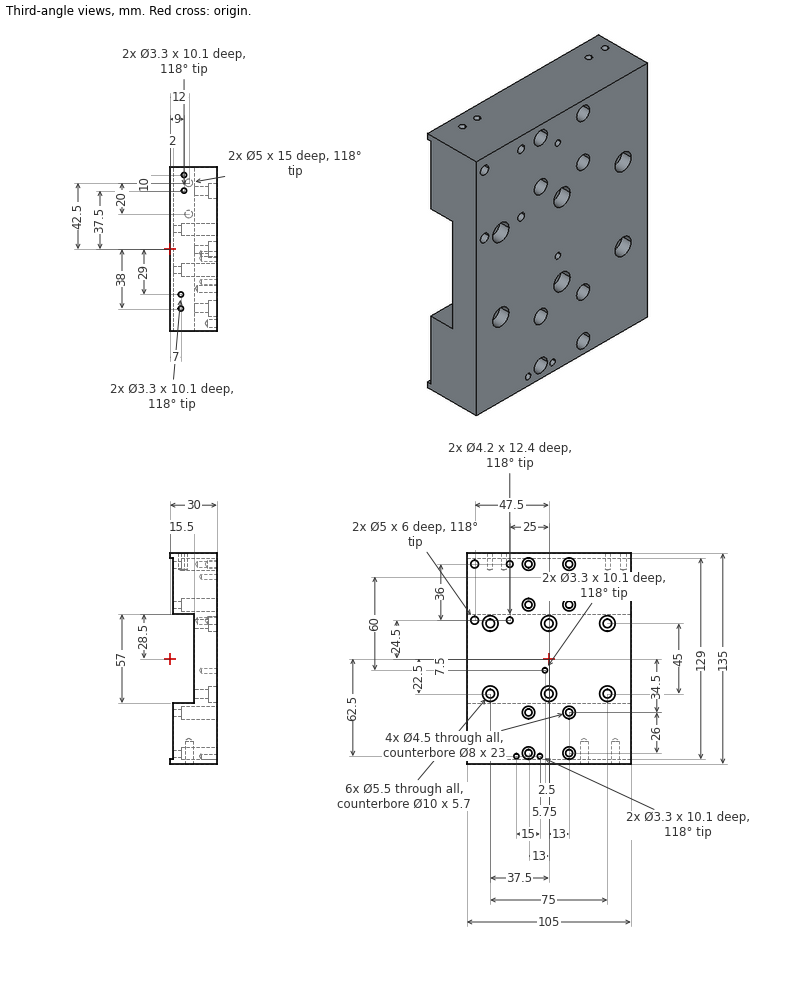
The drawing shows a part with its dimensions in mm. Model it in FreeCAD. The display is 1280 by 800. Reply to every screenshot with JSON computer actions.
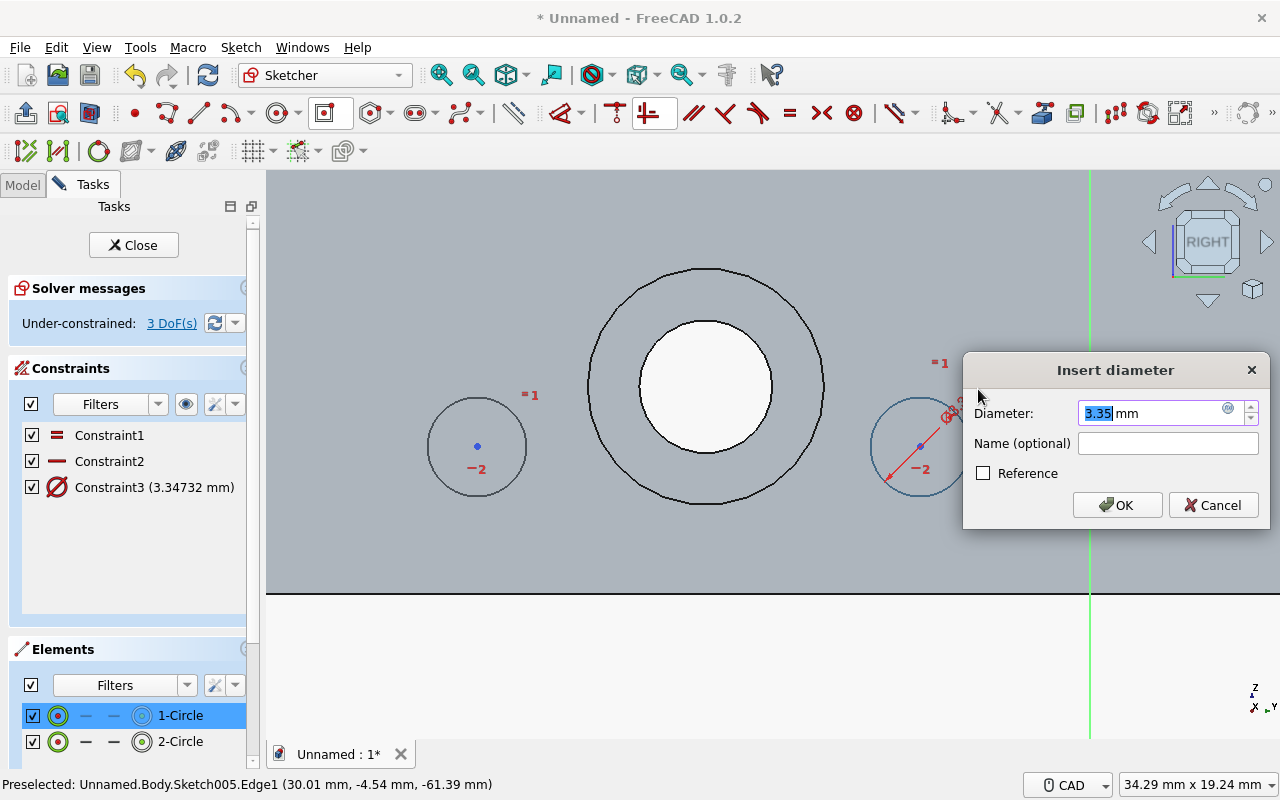
{"action": "type", "text": "3.3"}
{"action": "key", "text": "Return"}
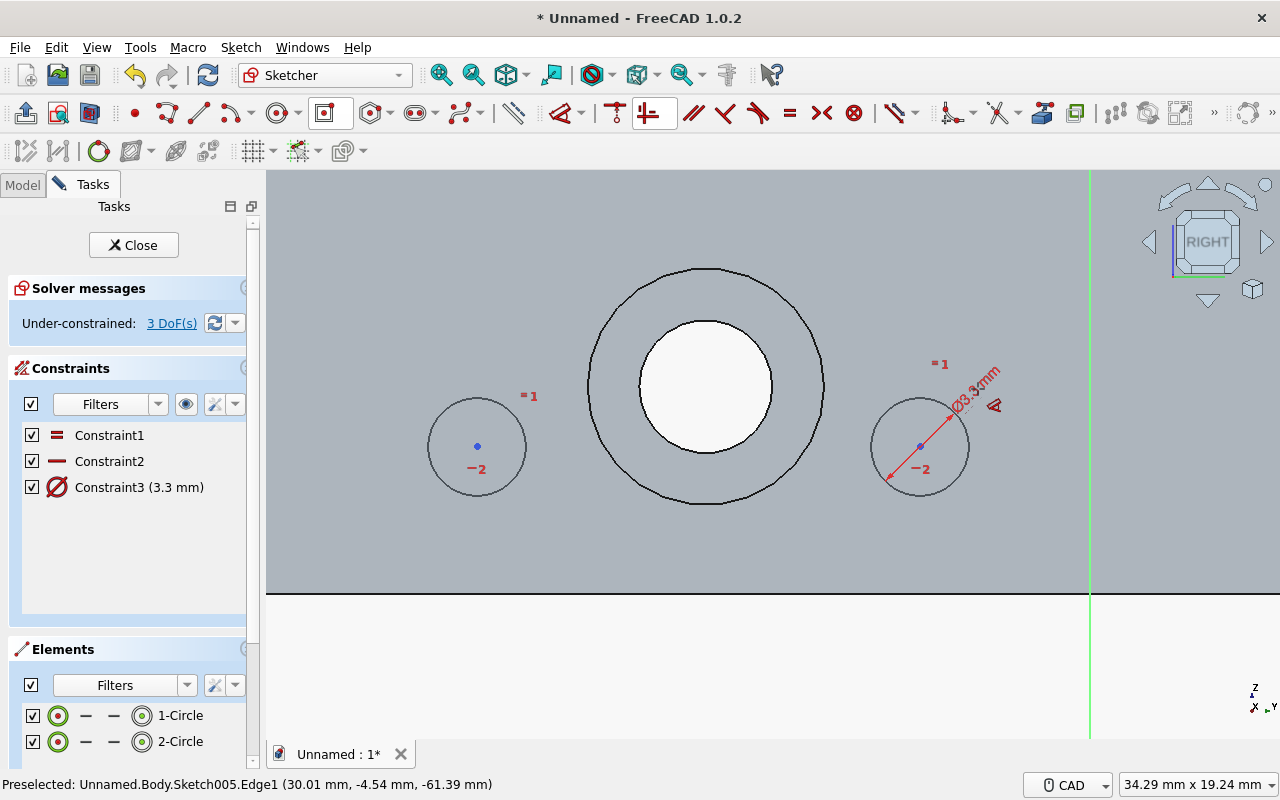
{"action": "left_click", "coordinate": [920, 447]}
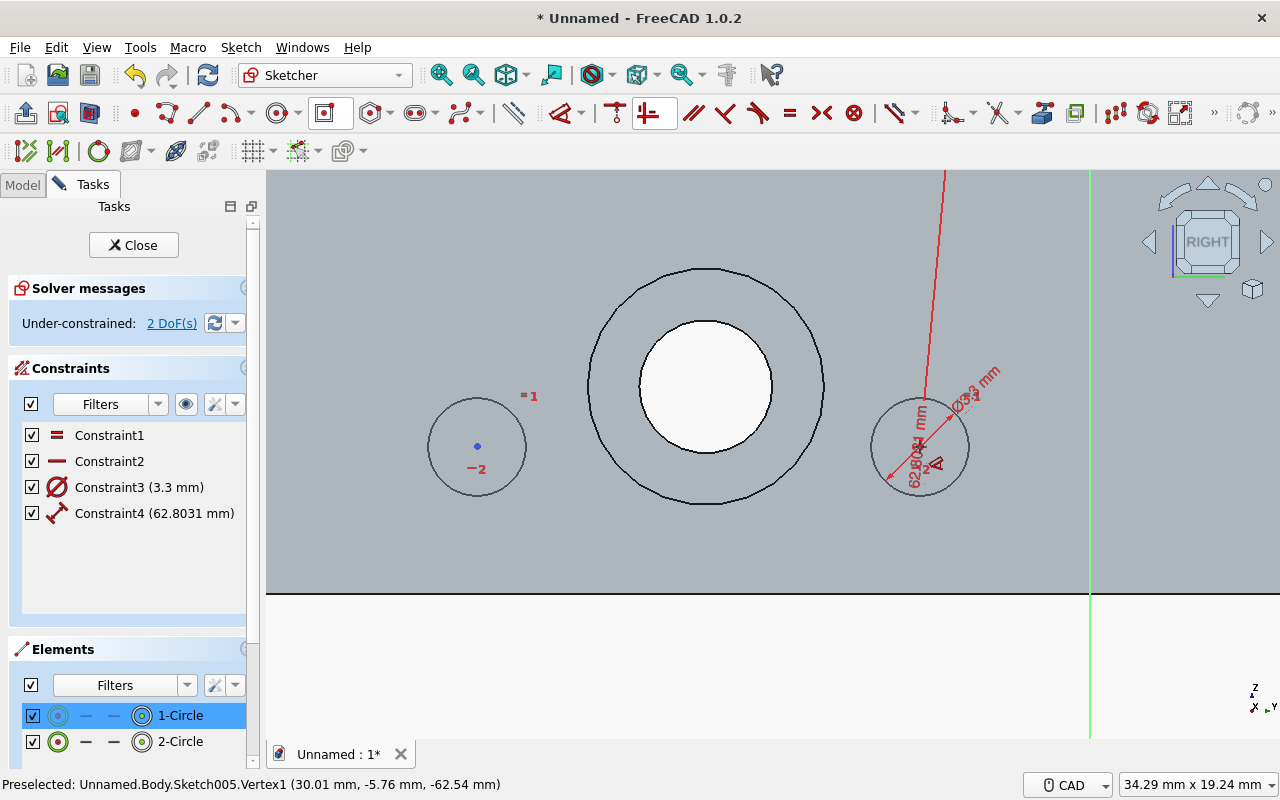
{"action": "left_click", "coordinate": [477, 447]}
{"action": "left_click", "coordinate": [699, 481]}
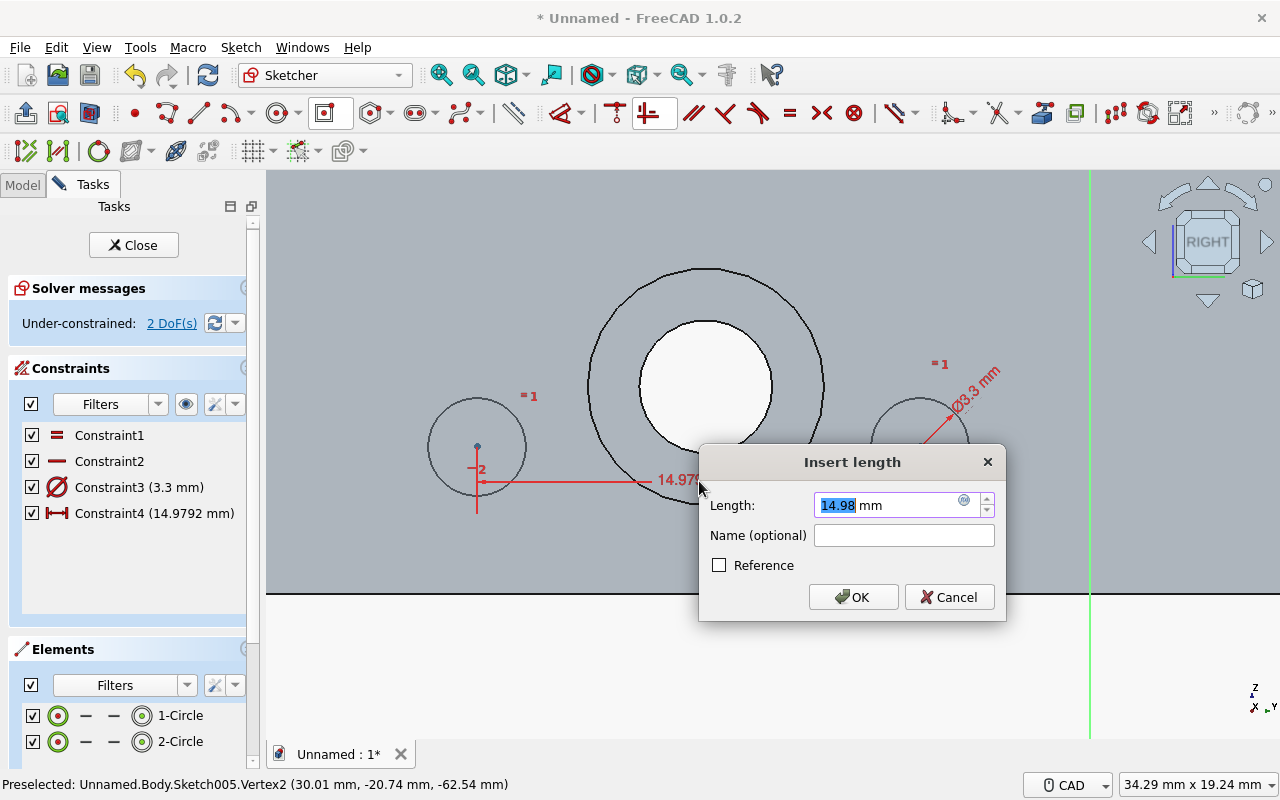
{"action": "type", "text": "15"}
{"action": "key", "text": "Return"}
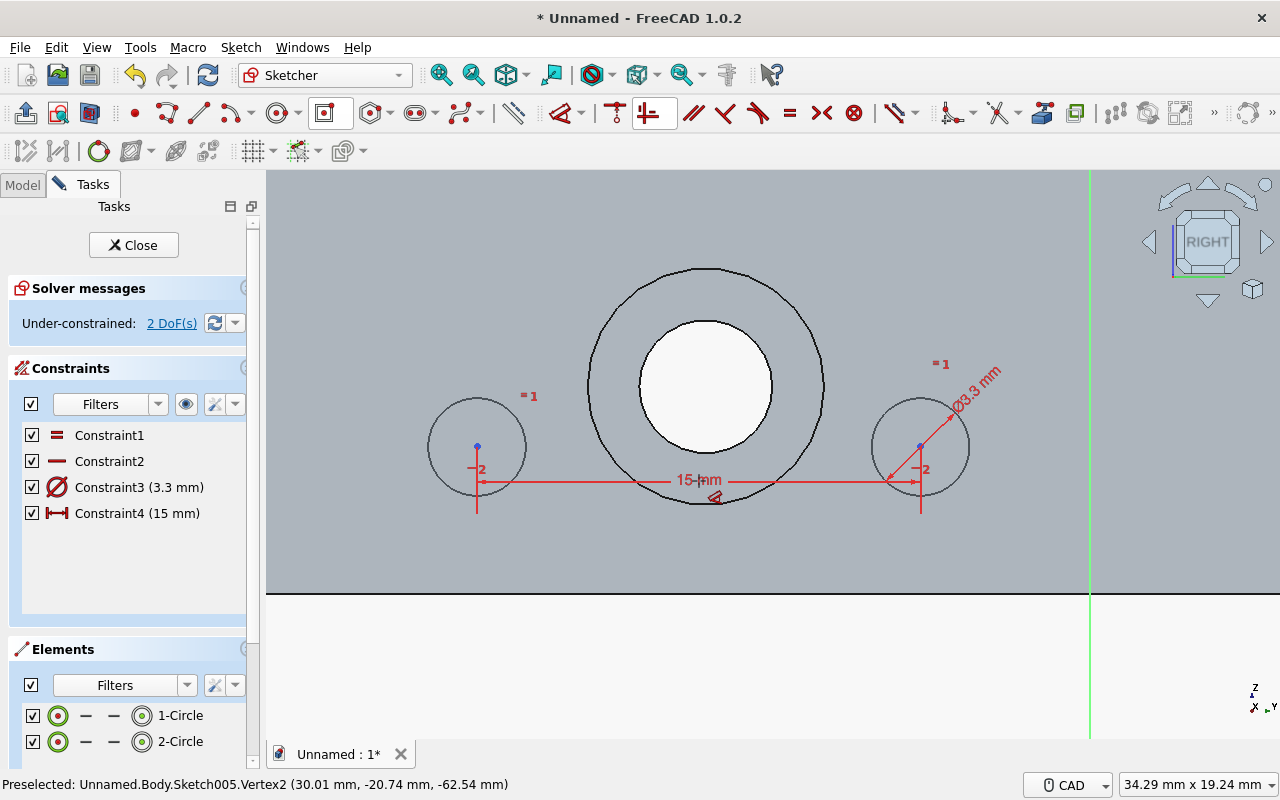
{"action": "left_click", "coordinate": [921, 447]}
{"action": "left_click", "coordinate": [1005, 481]}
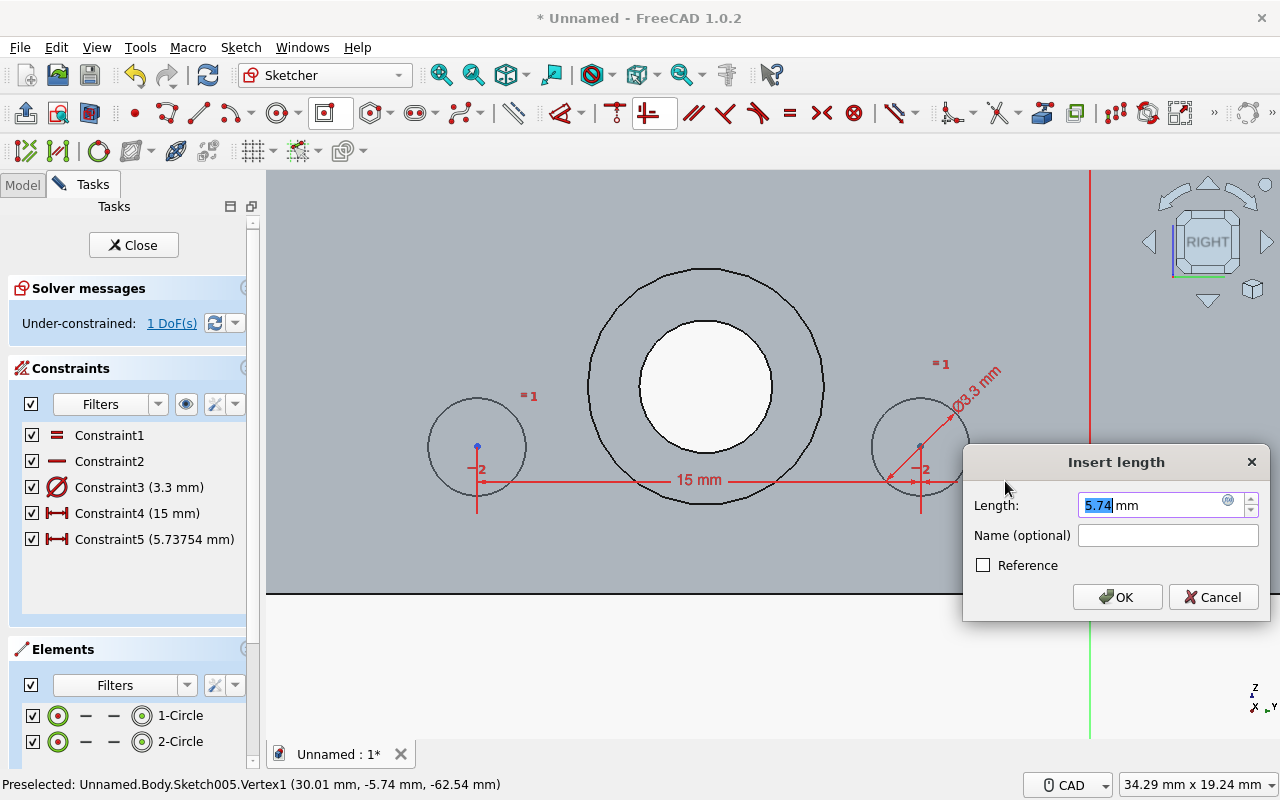
{"action": "type", "text": "5.75"}
{"action": "key", "text": "Return"}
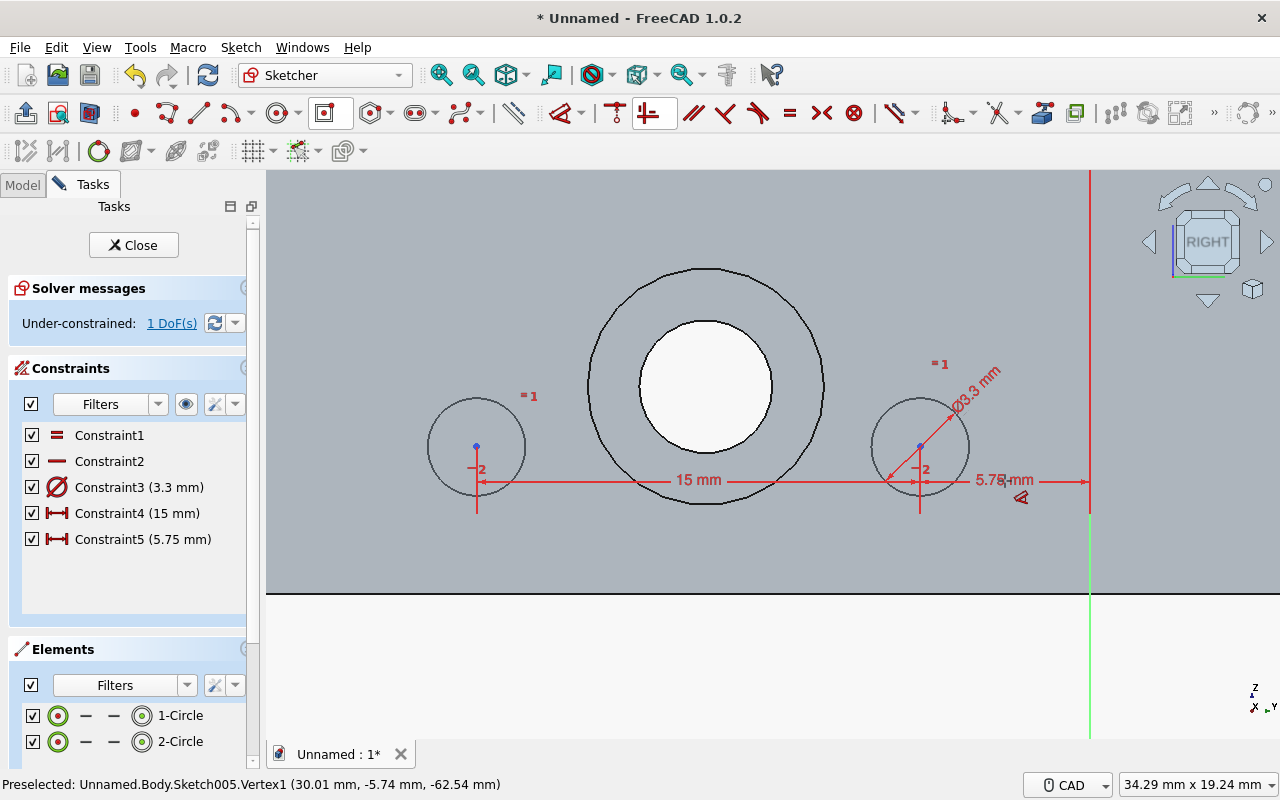
{"action": "left_click", "coordinate": [920, 447]}
{"action": "left_click", "coordinate": [886, 322]}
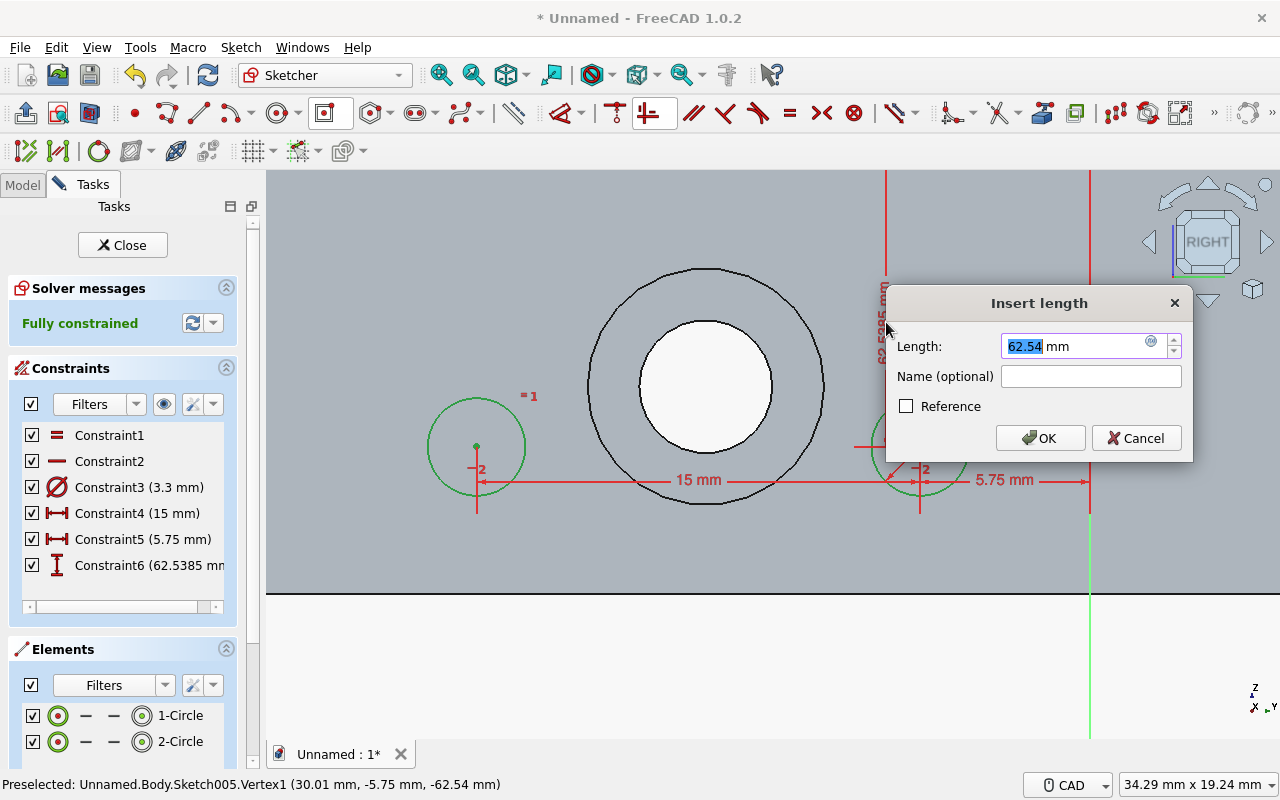
{"action": "type", "text": "62.5"}
{"action": "key", "text": "Return"}
{"action": "key", "text": "Escape"}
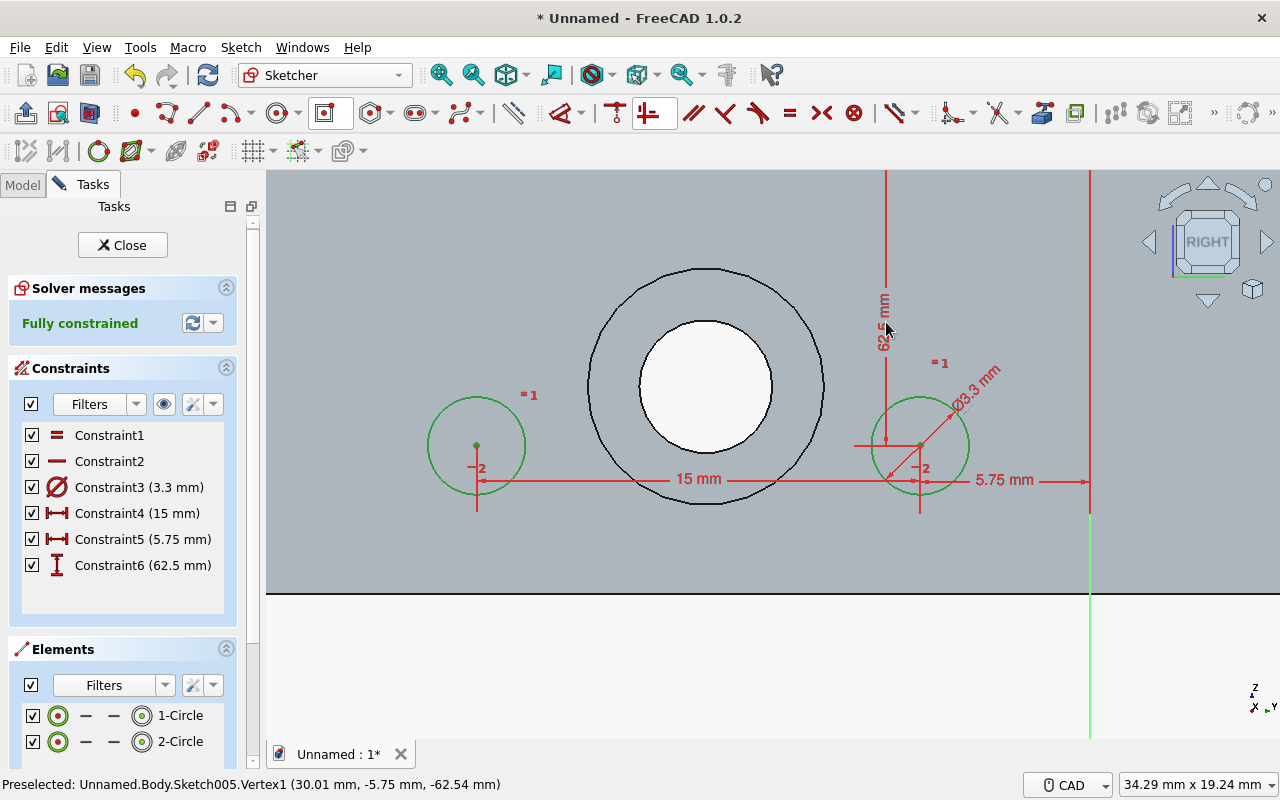
{"action": "left_click", "coordinate": [123, 245]}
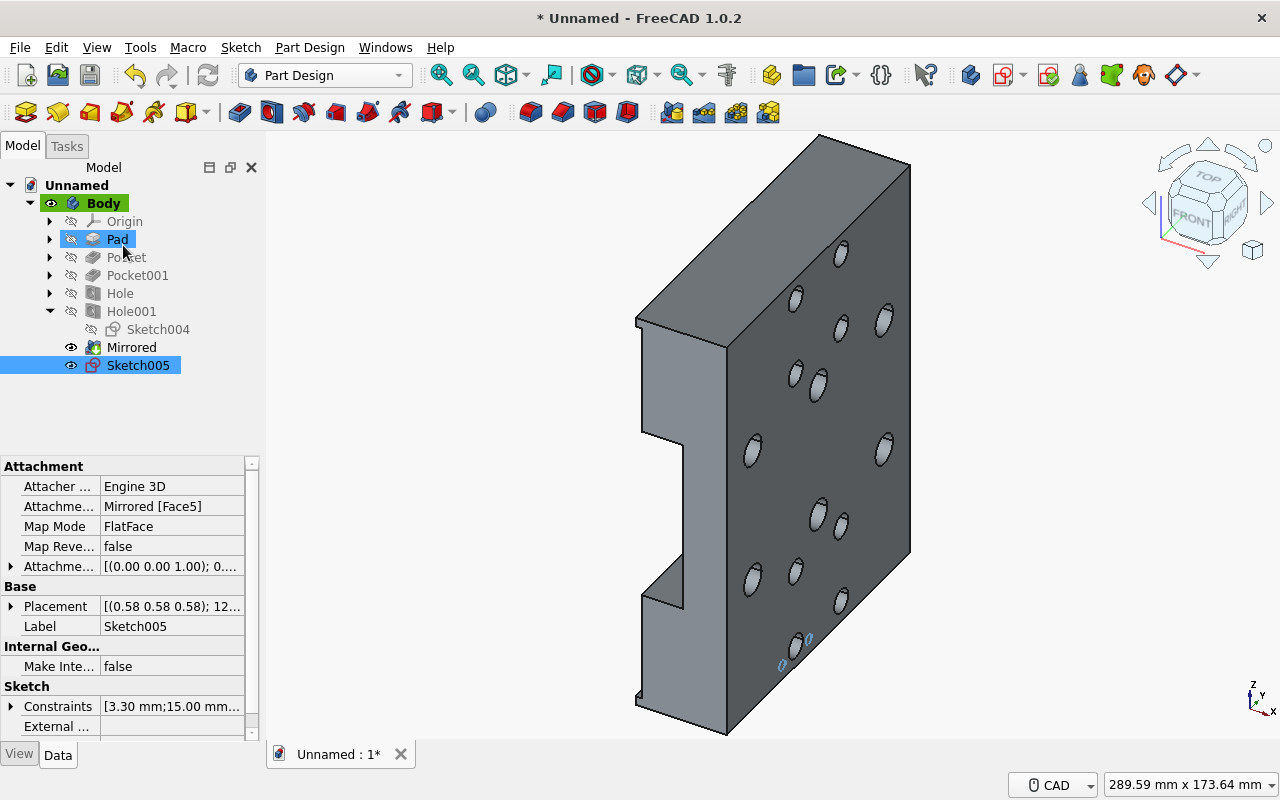
{"action": "left_click", "coordinate": [272, 112]}